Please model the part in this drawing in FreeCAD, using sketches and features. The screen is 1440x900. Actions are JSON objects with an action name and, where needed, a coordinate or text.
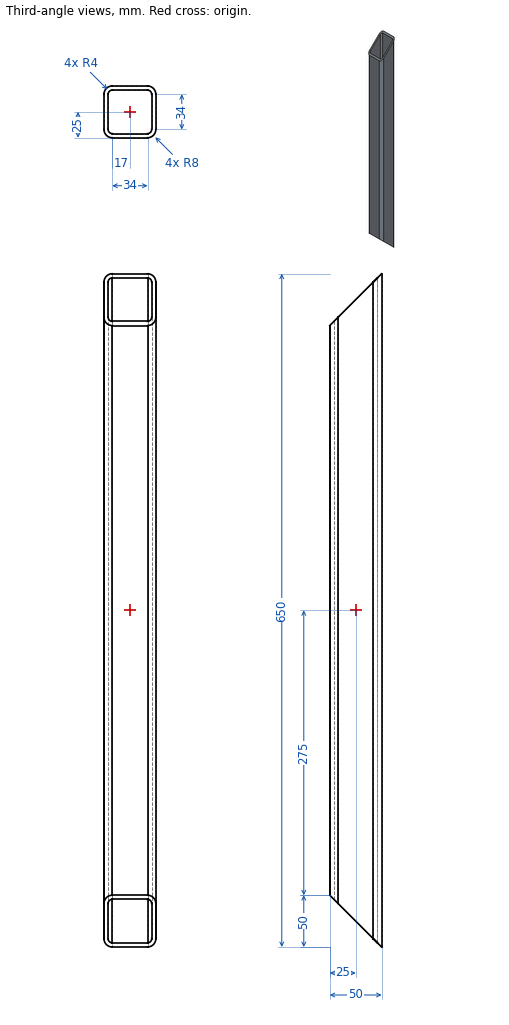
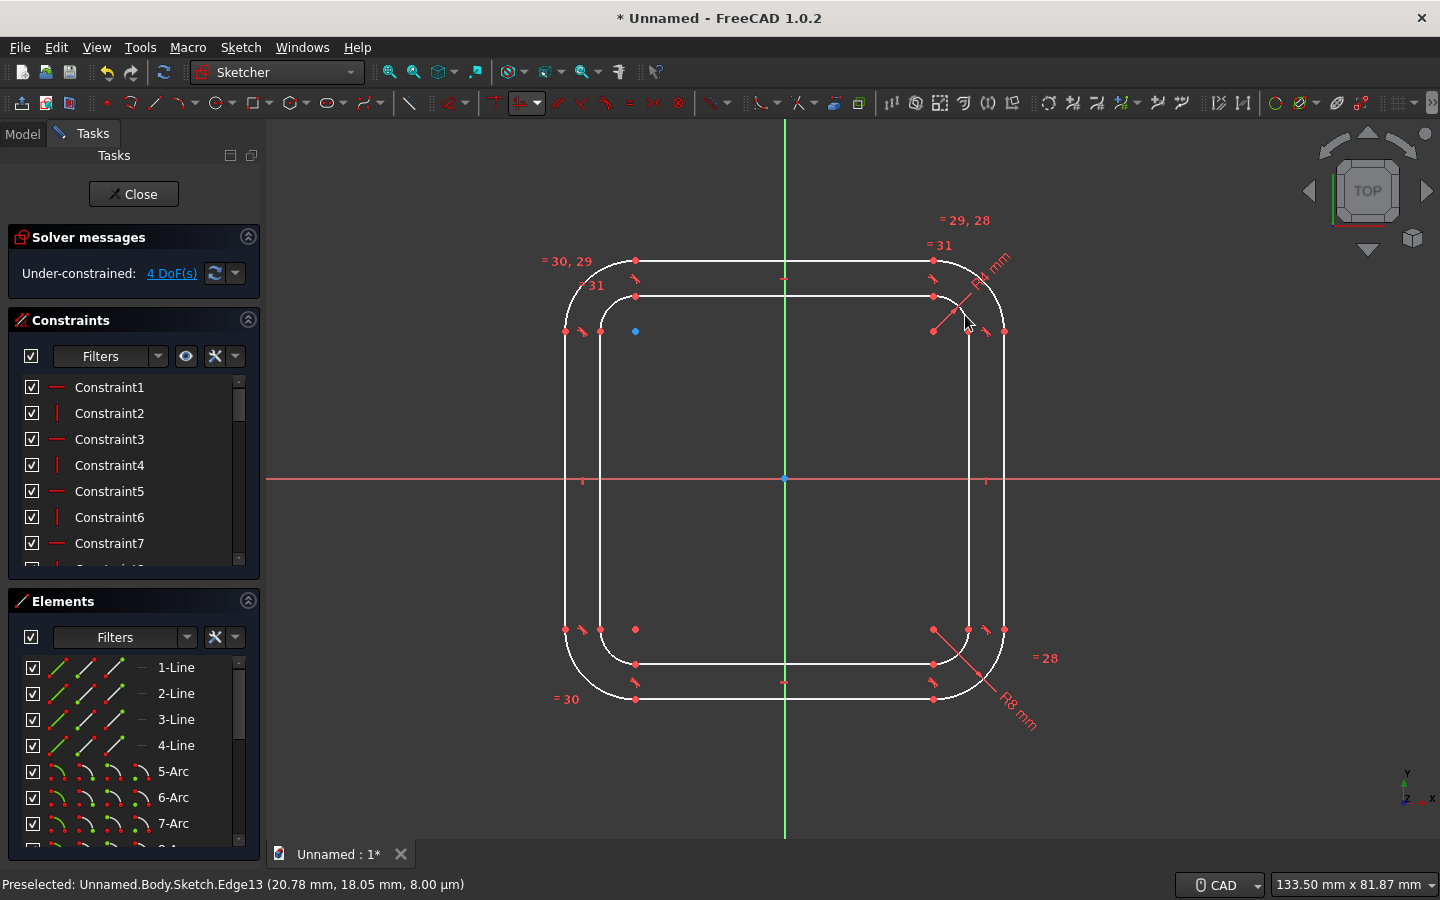
{"action": "left_click", "coordinate": [725, 699]}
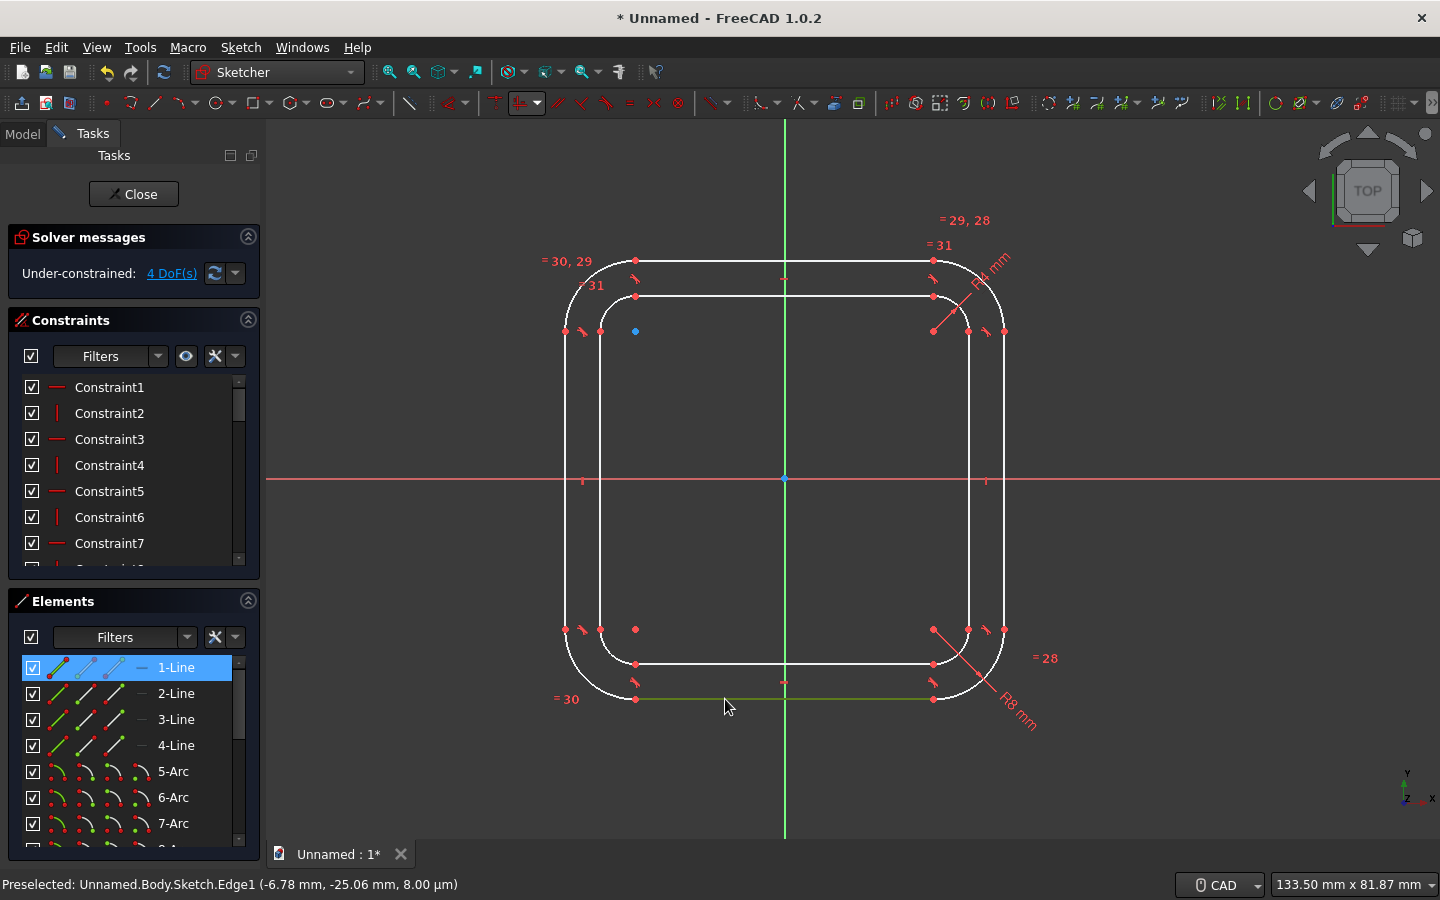
{"action": "left_click", "coordinate": [468, 104]}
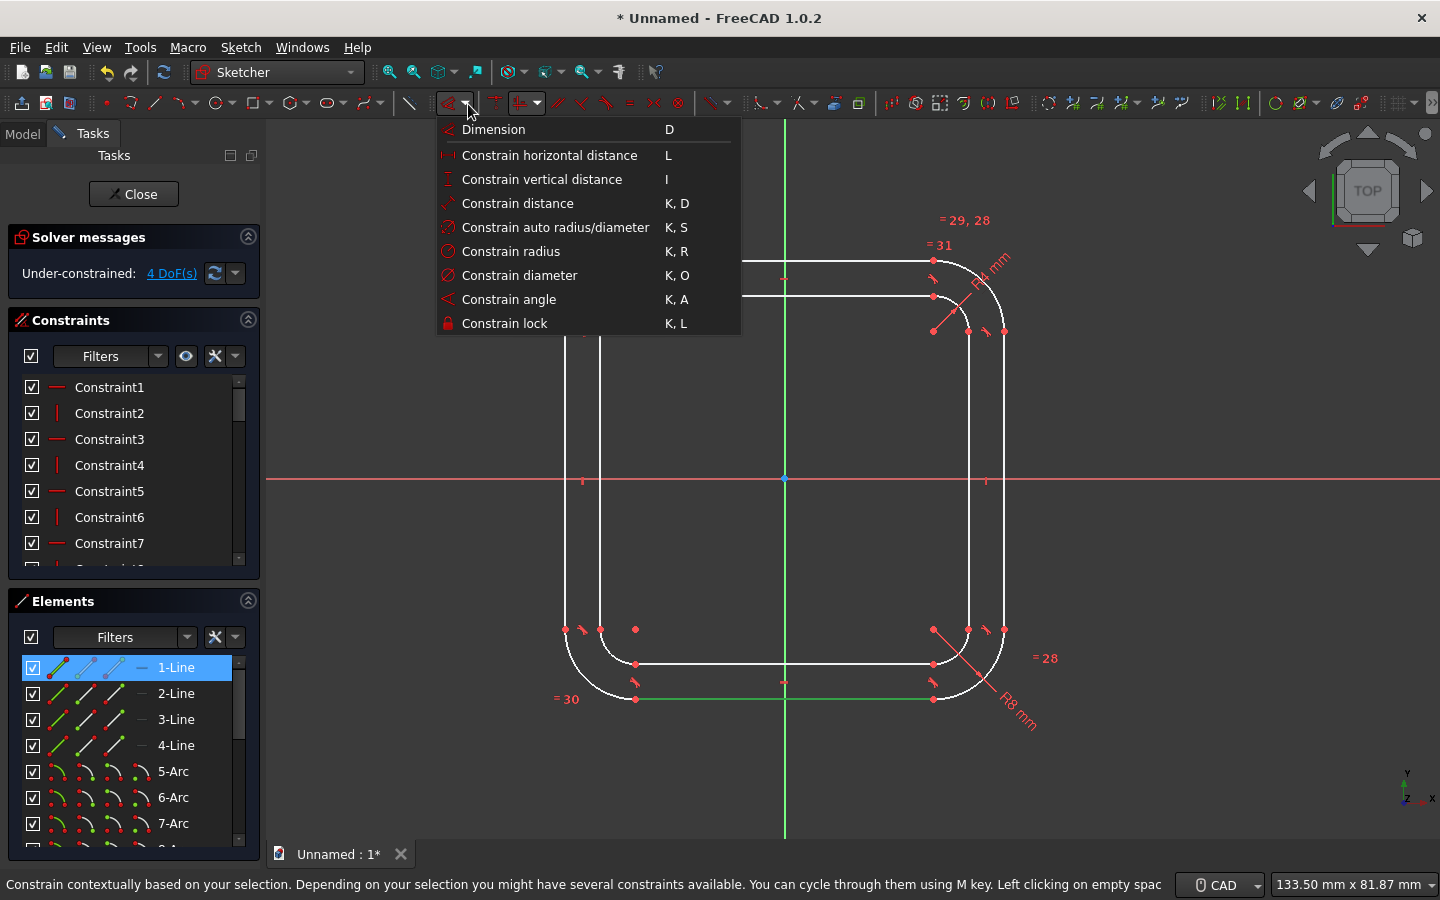
{"action": "left_click", "coordinate": [589, 155]}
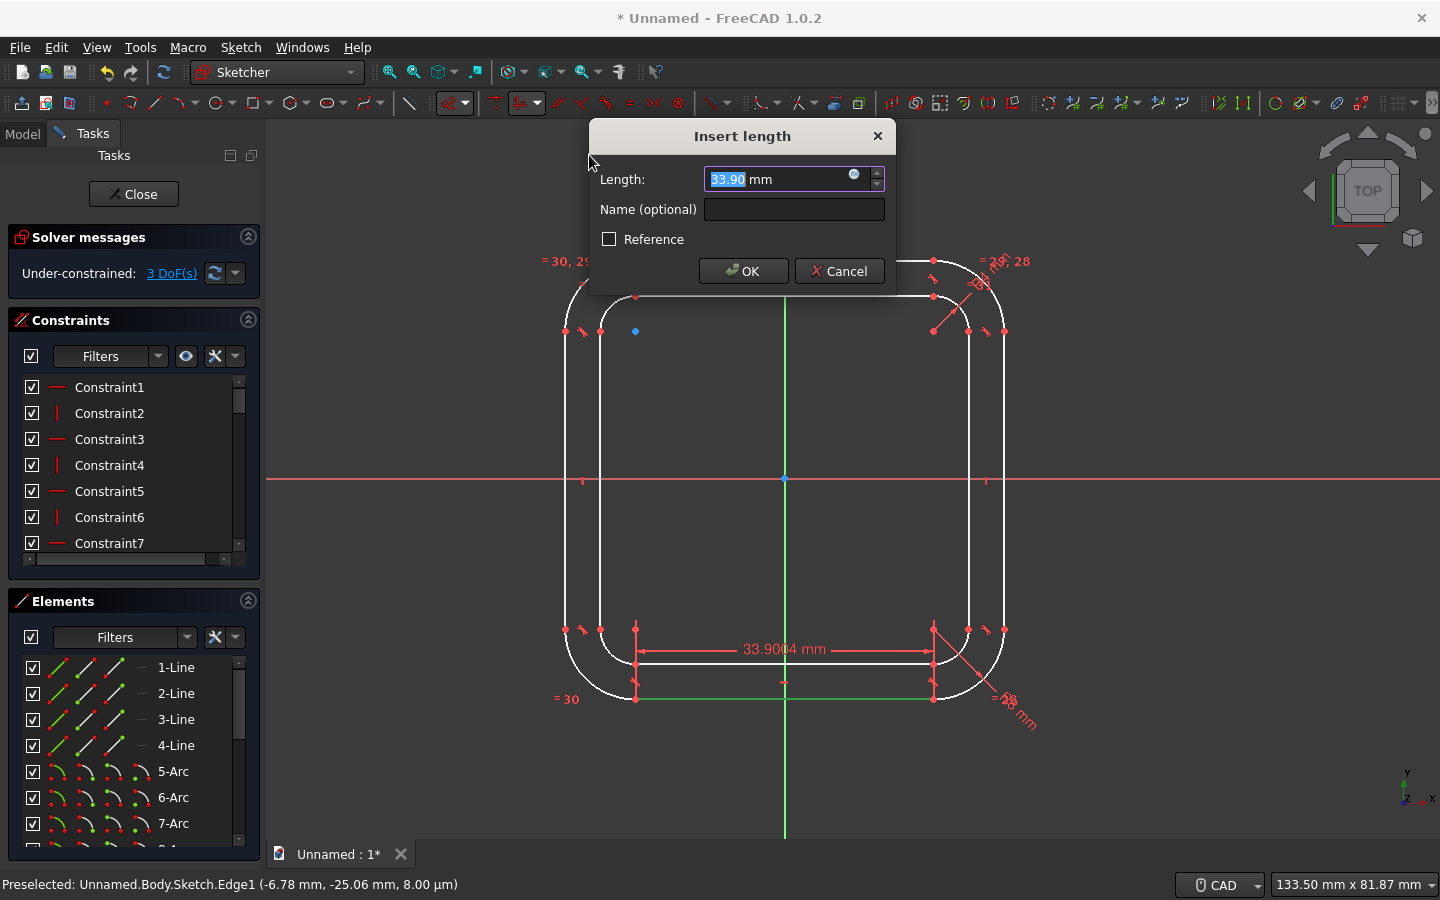
{"action": "type", "text": "34"}
{"action": "key", "text": "Return"}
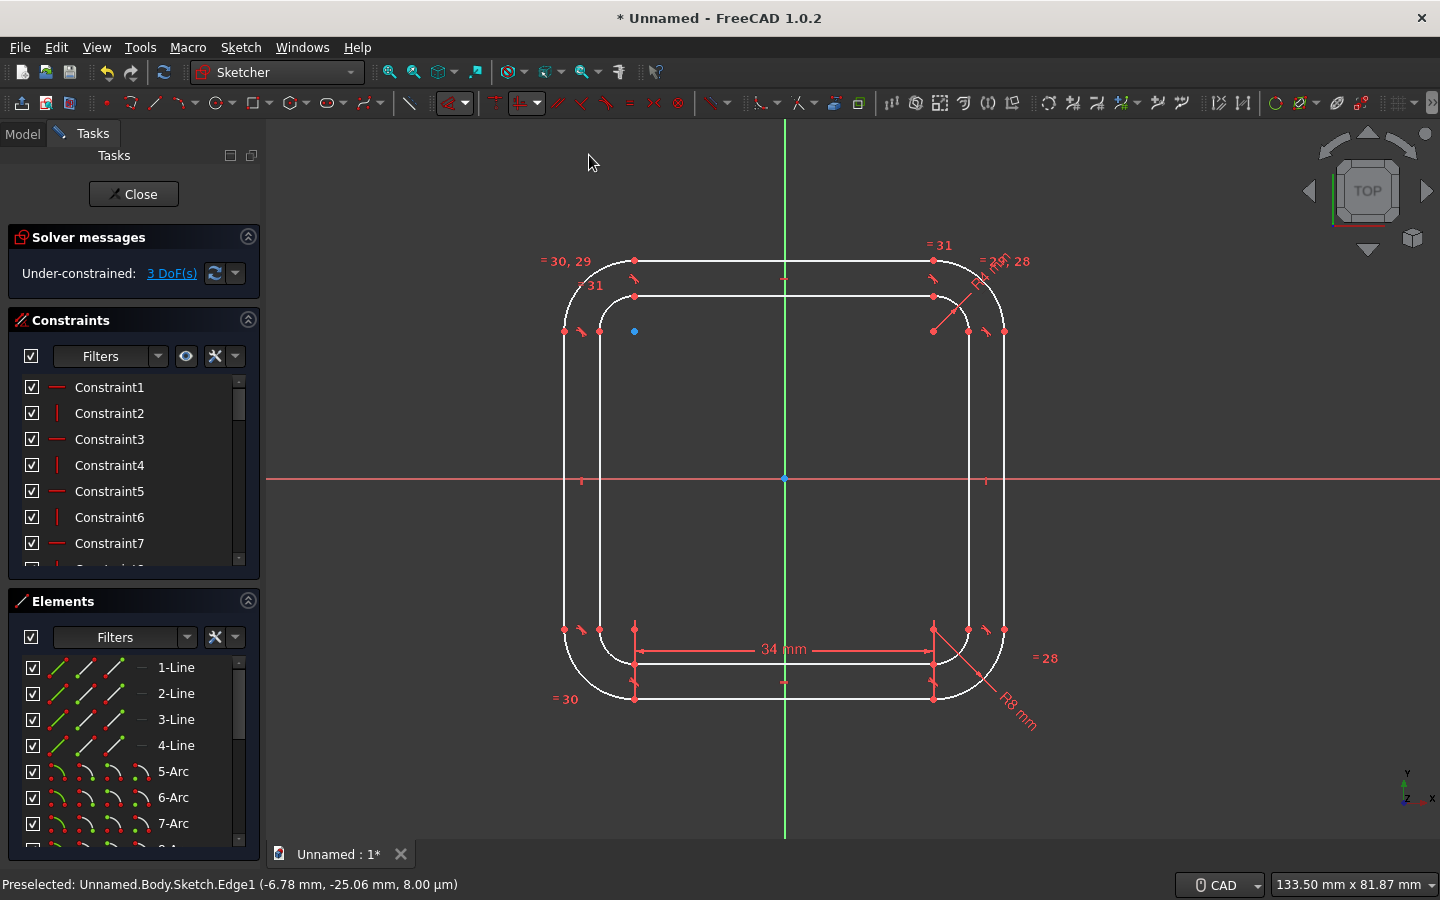
{"action": "left_click", "coordinate": [1004, 540]}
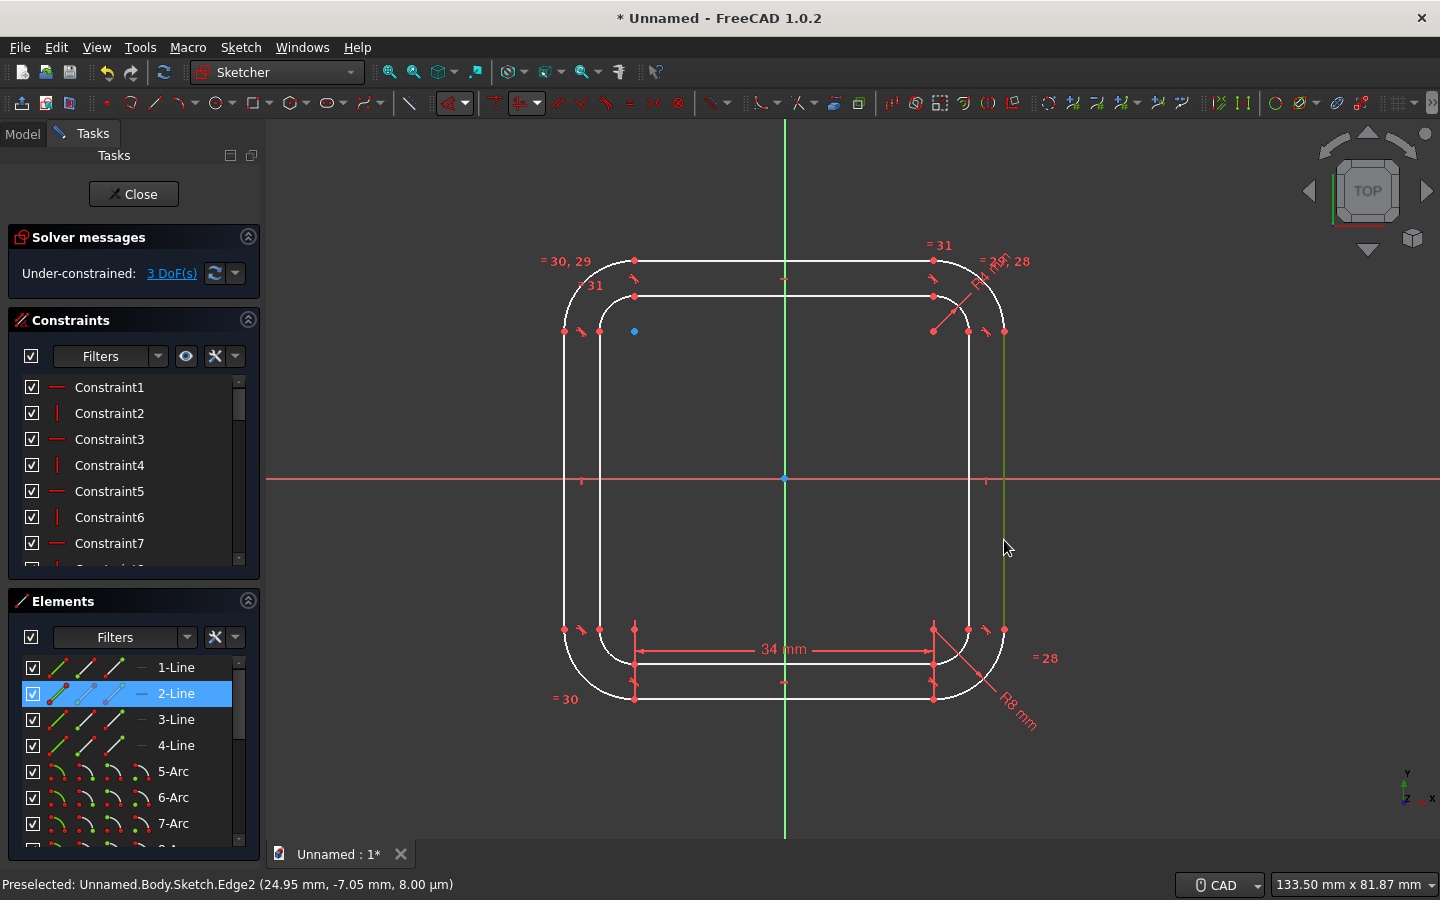
{"action": "key", "text": "i"}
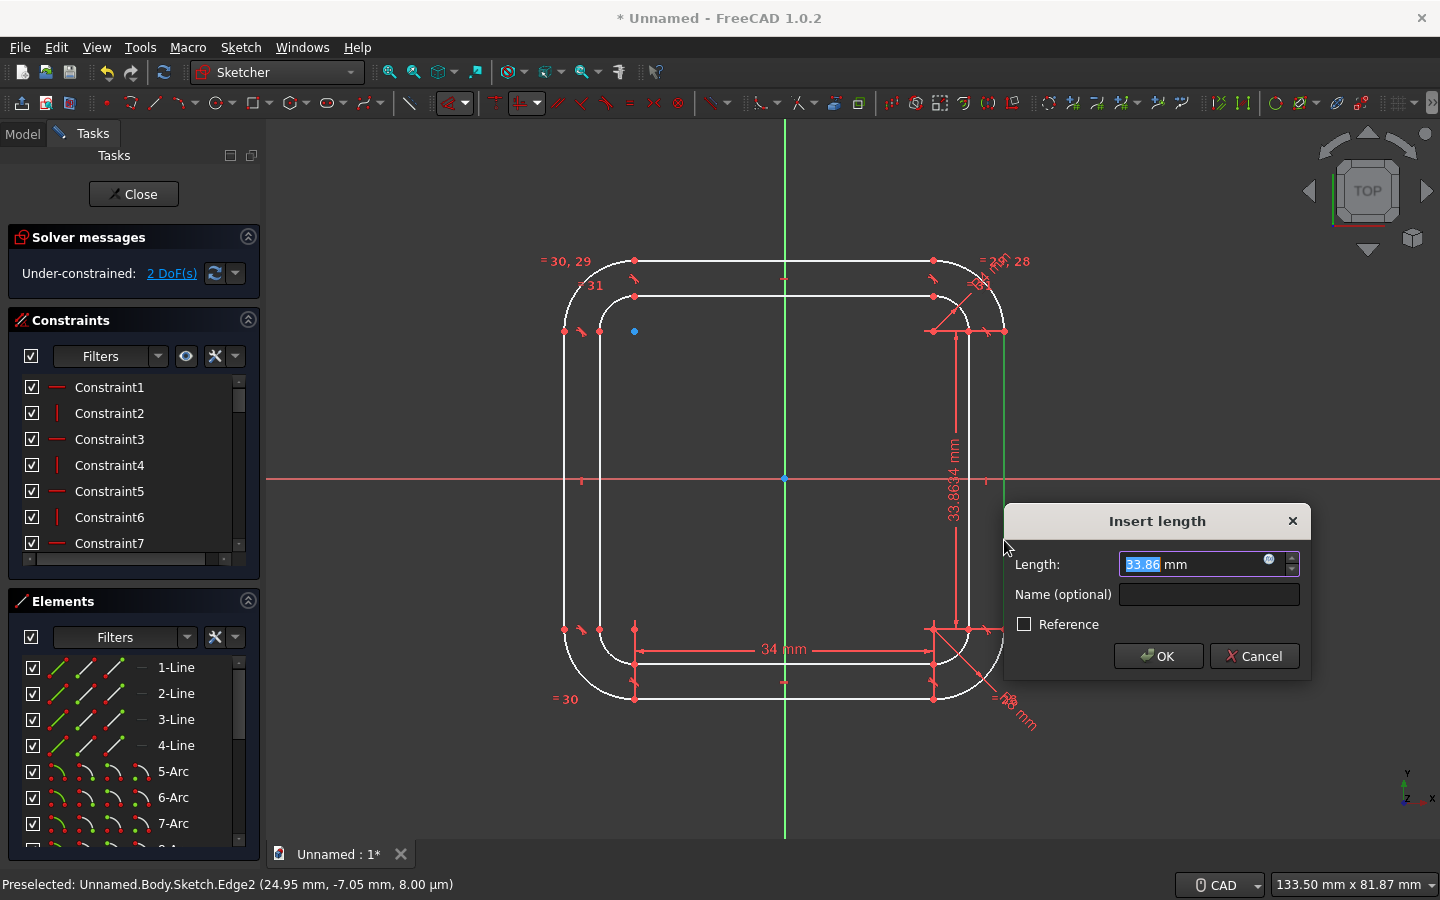
{"action": "type", "text": "34"}
{"action": "key", "text": "Return"}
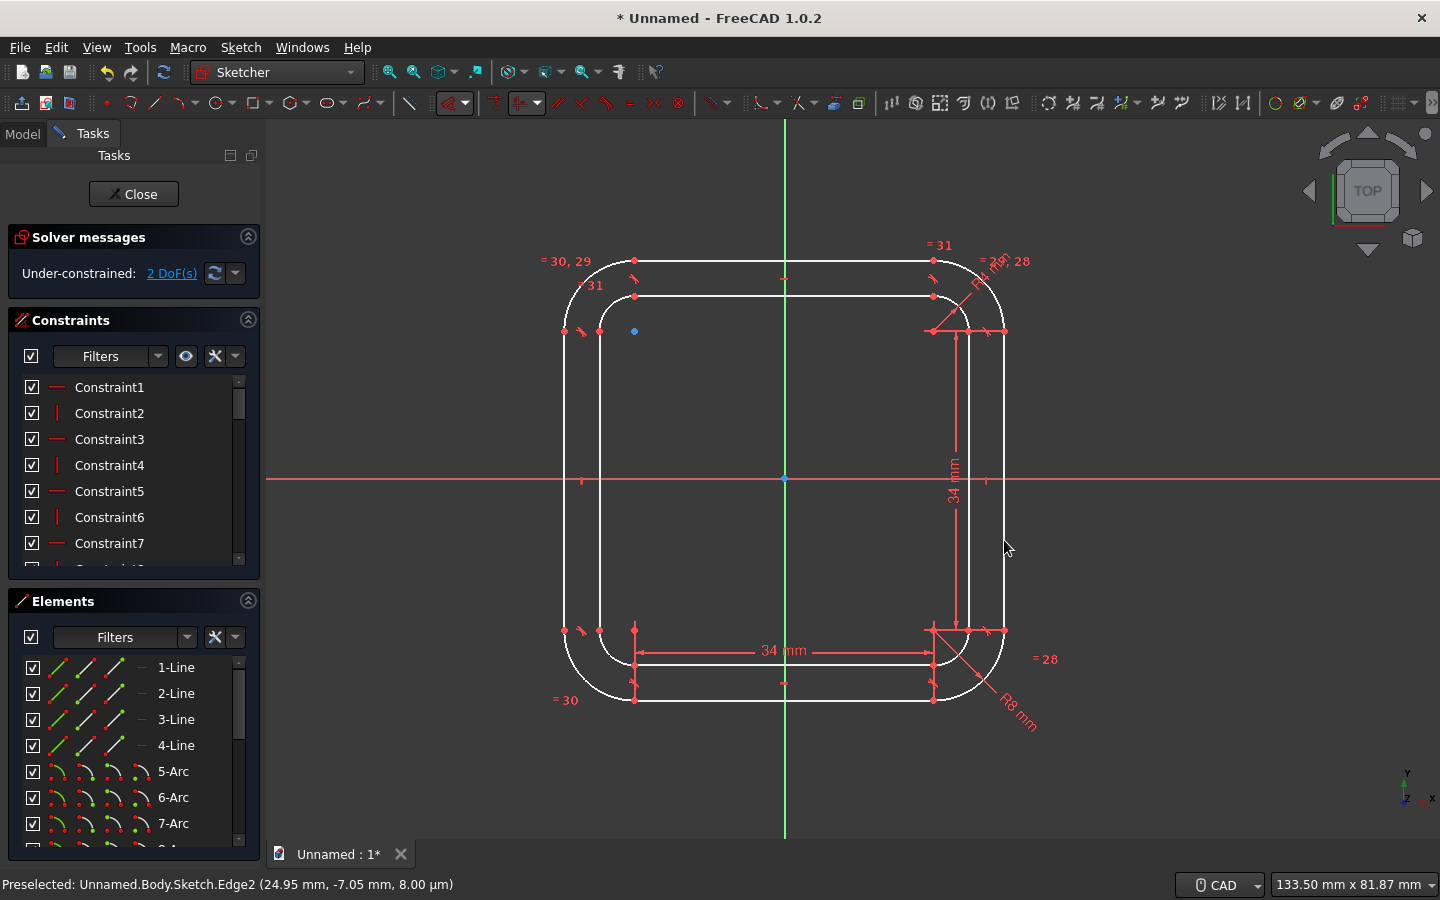
{"action": "left_click", "coordinate": [635, 701]}